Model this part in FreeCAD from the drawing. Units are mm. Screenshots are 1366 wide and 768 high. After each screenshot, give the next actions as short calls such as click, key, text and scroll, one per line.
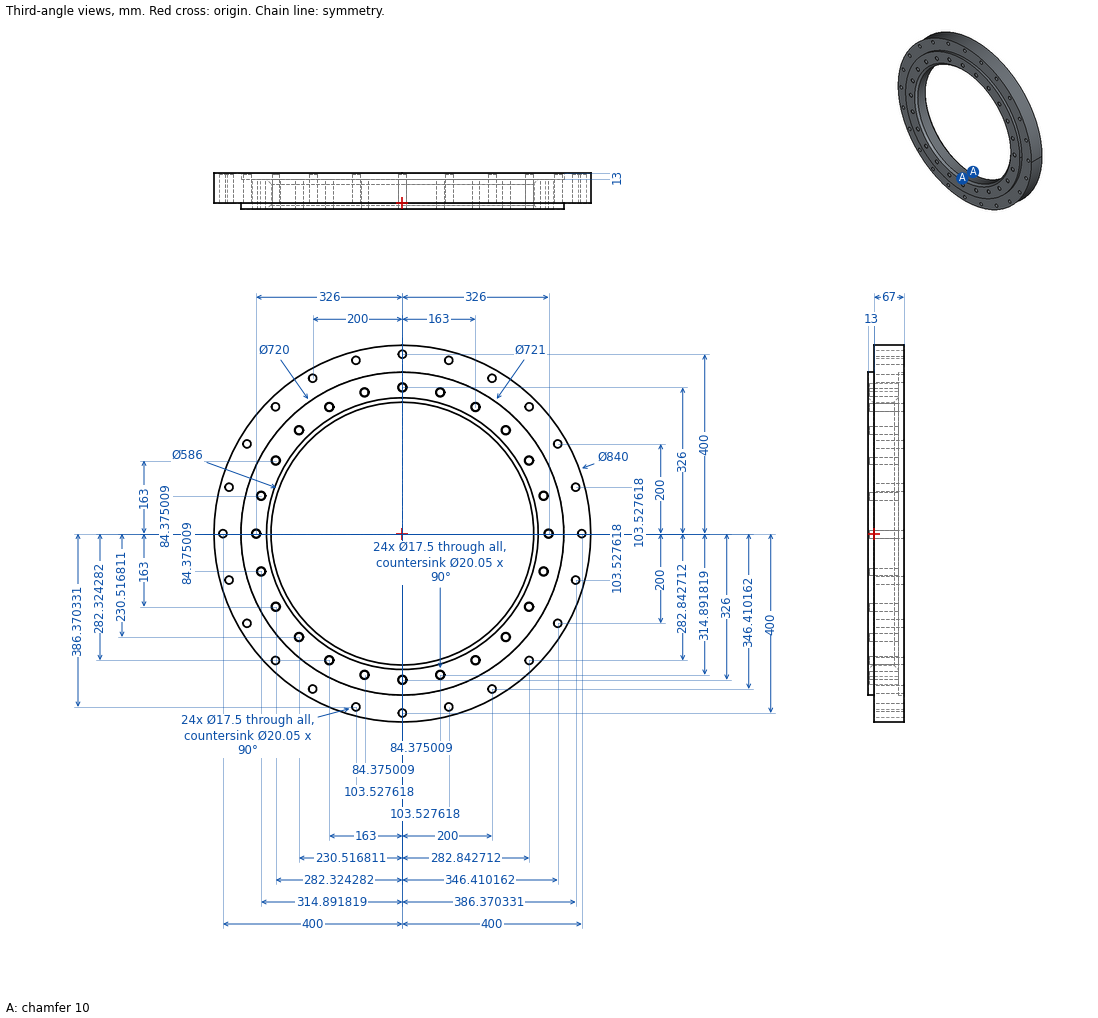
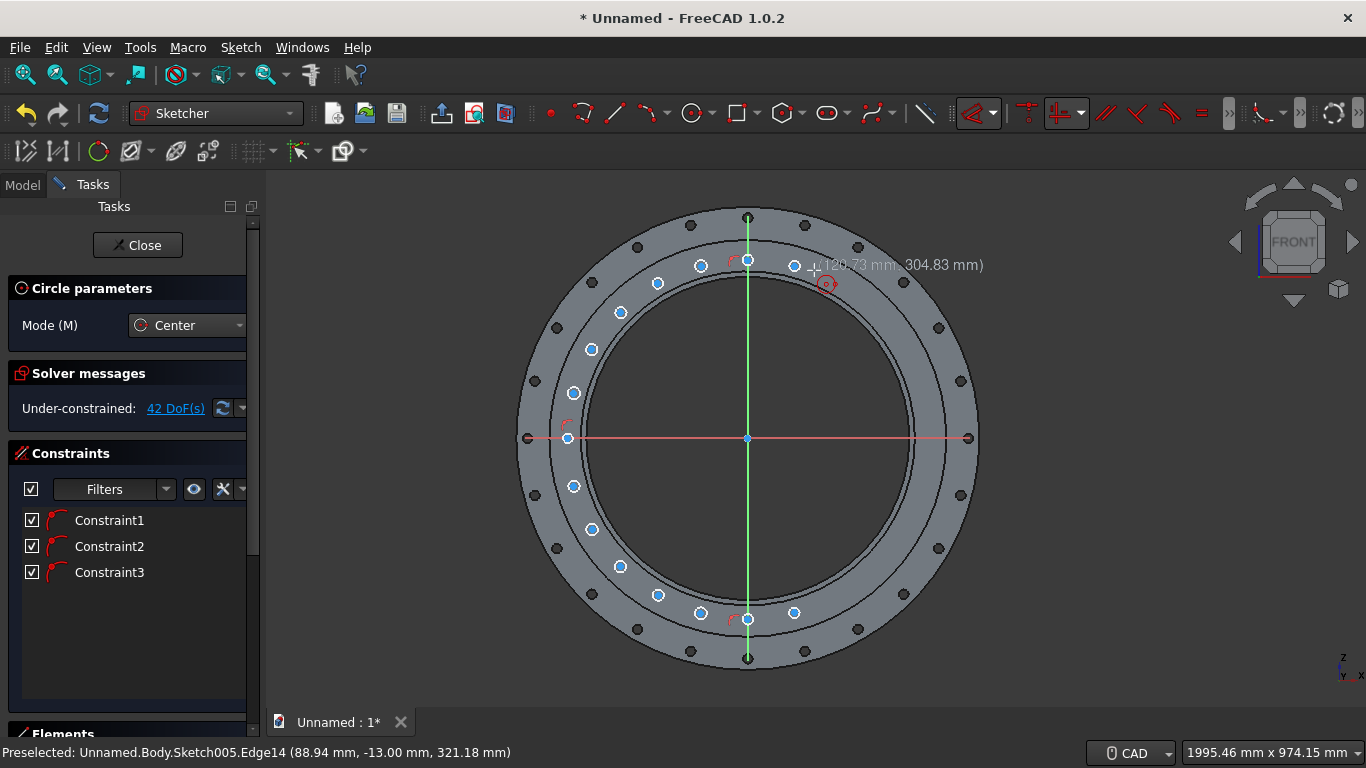
click(838, 283)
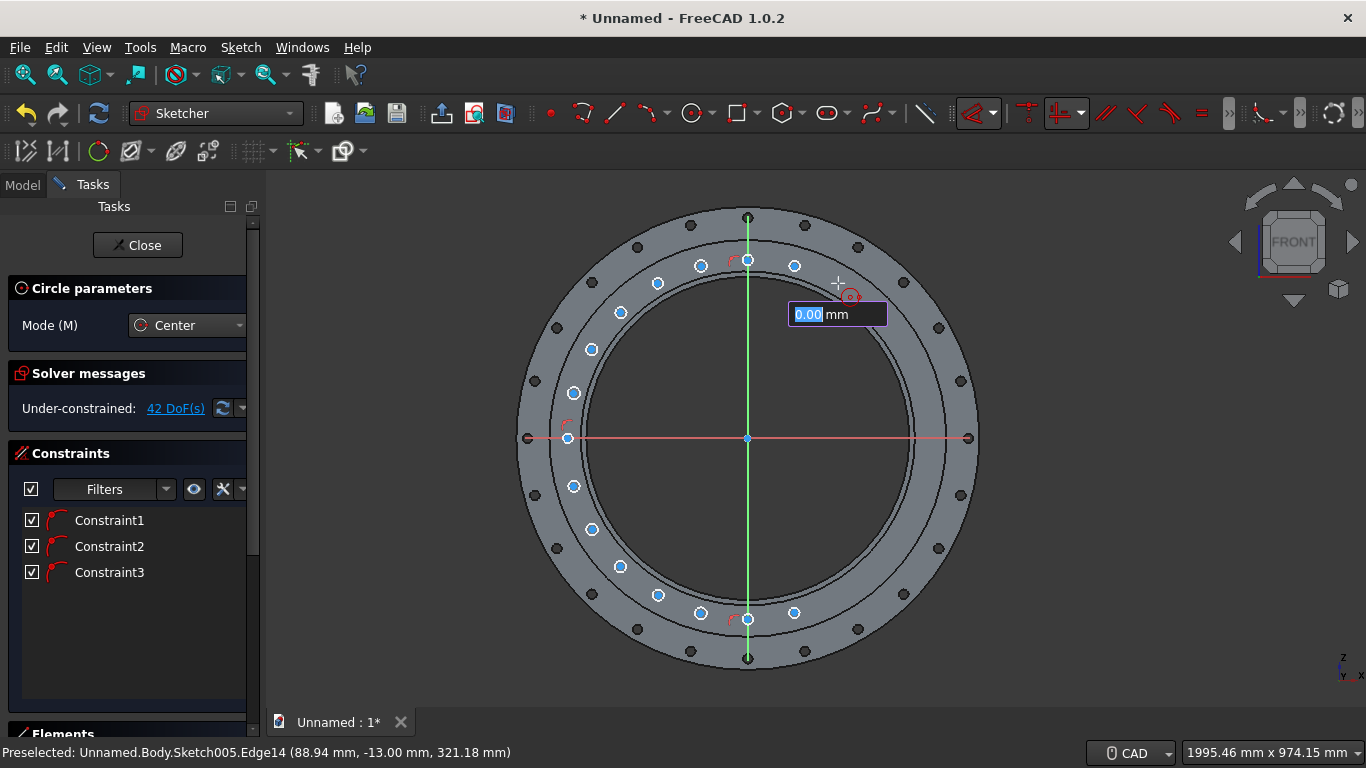
scroll(841, 279, up, 6)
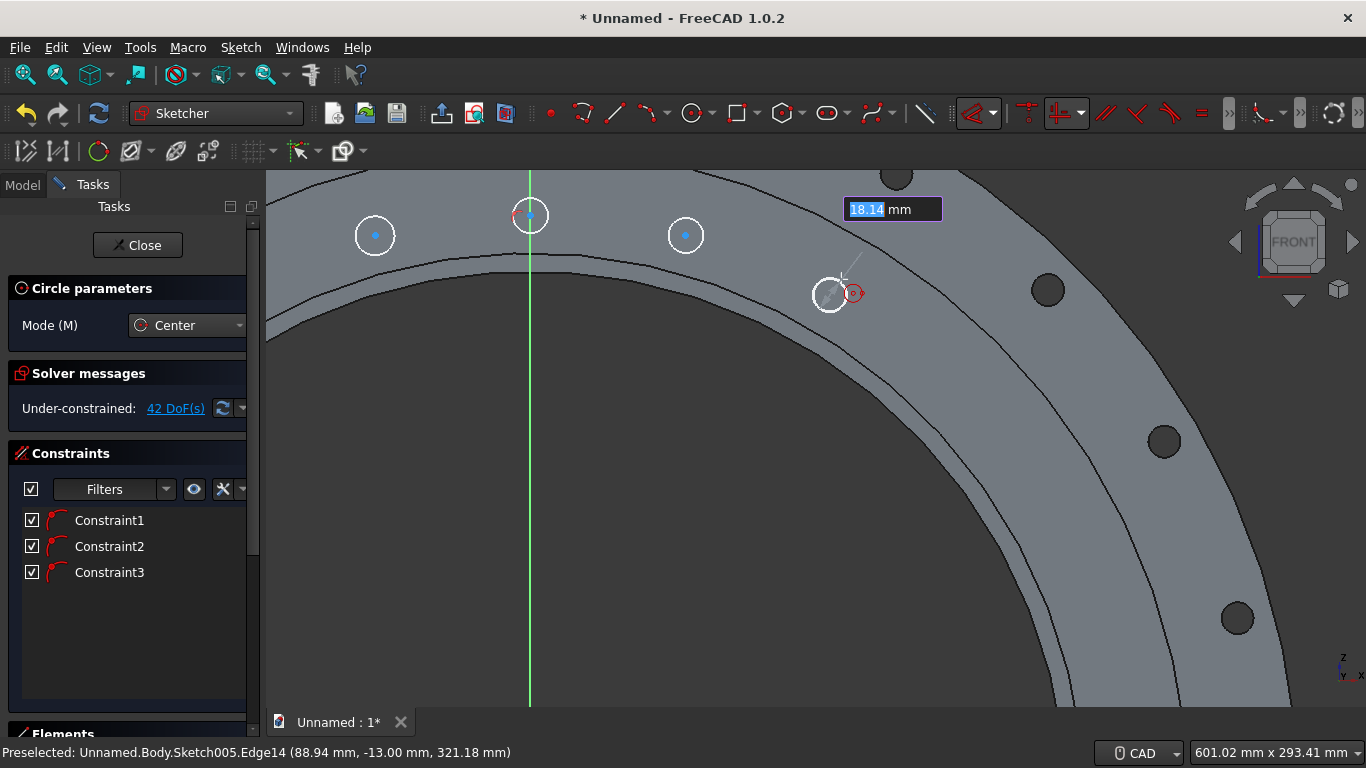
click(840, 280)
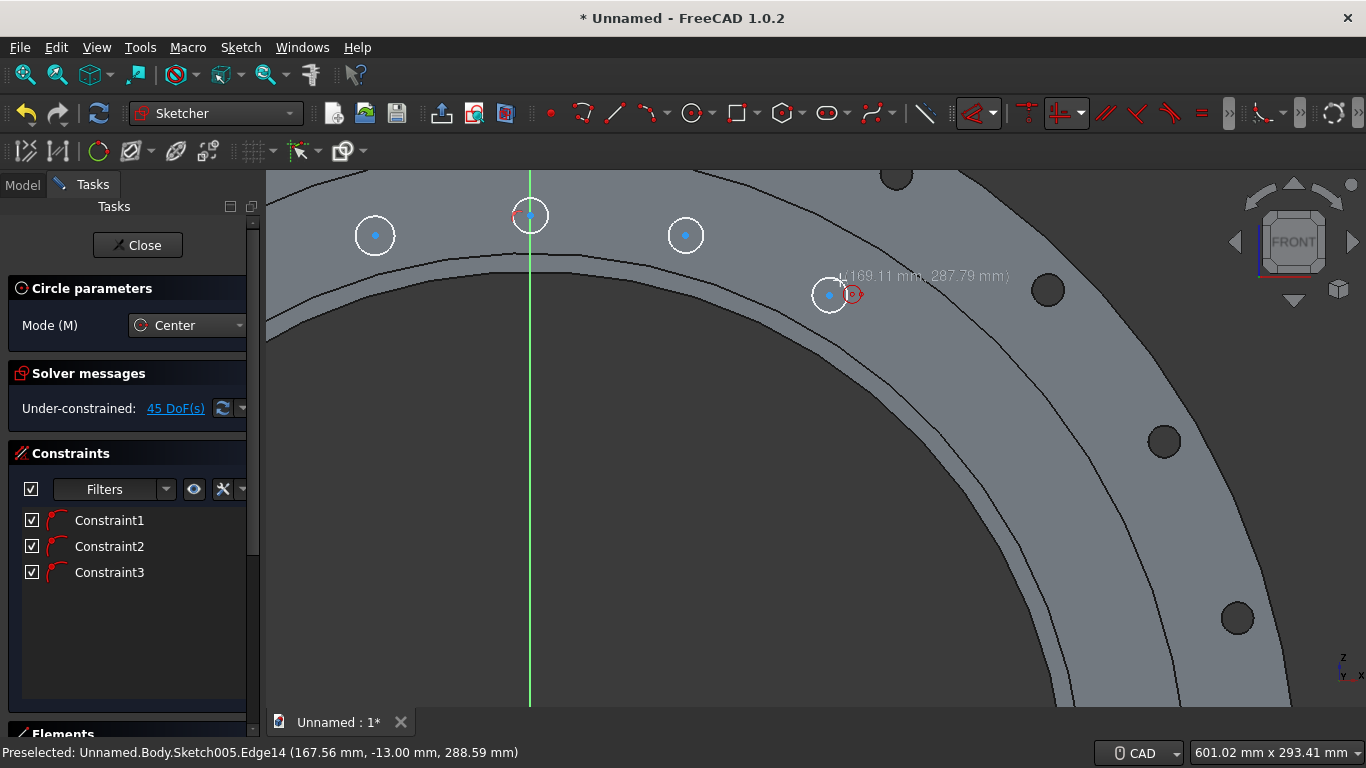
scroll(952, 386, up, 2)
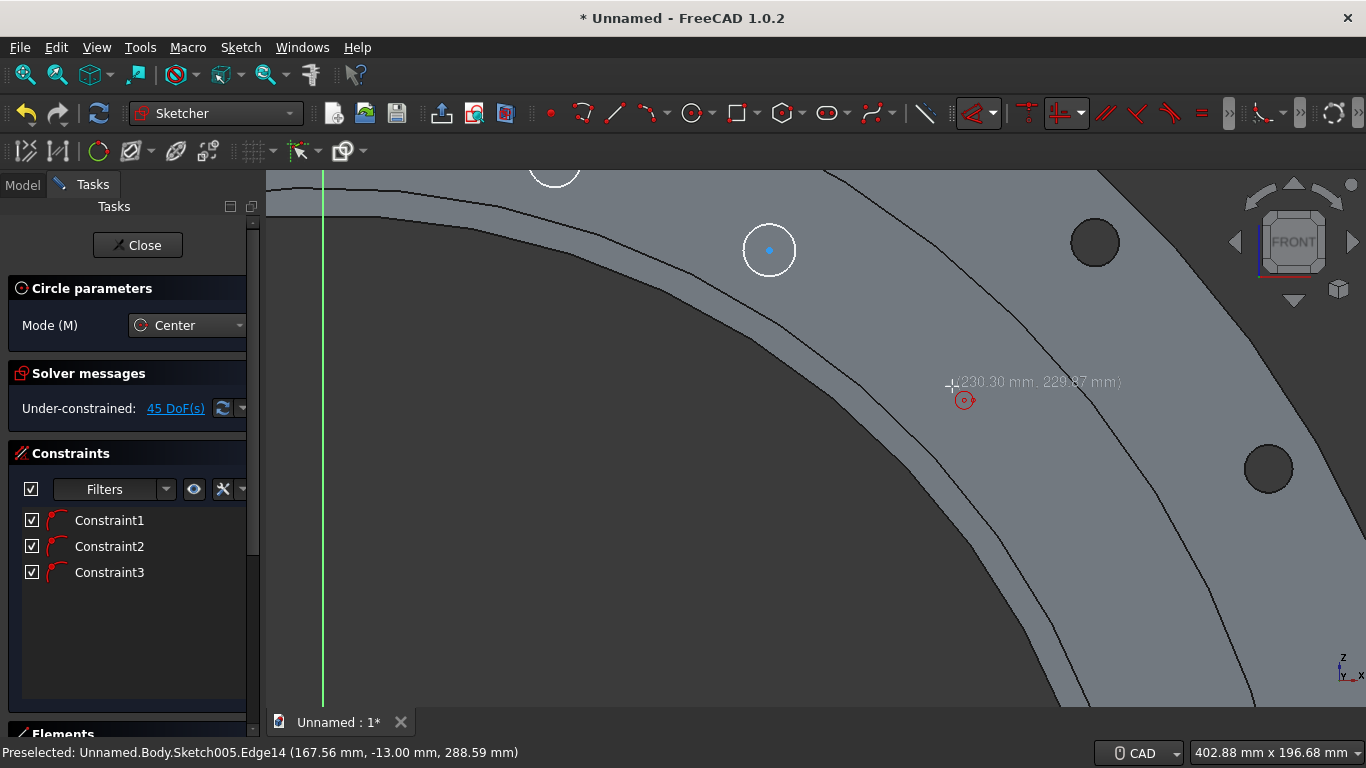
scroll(855, 293, down, 8)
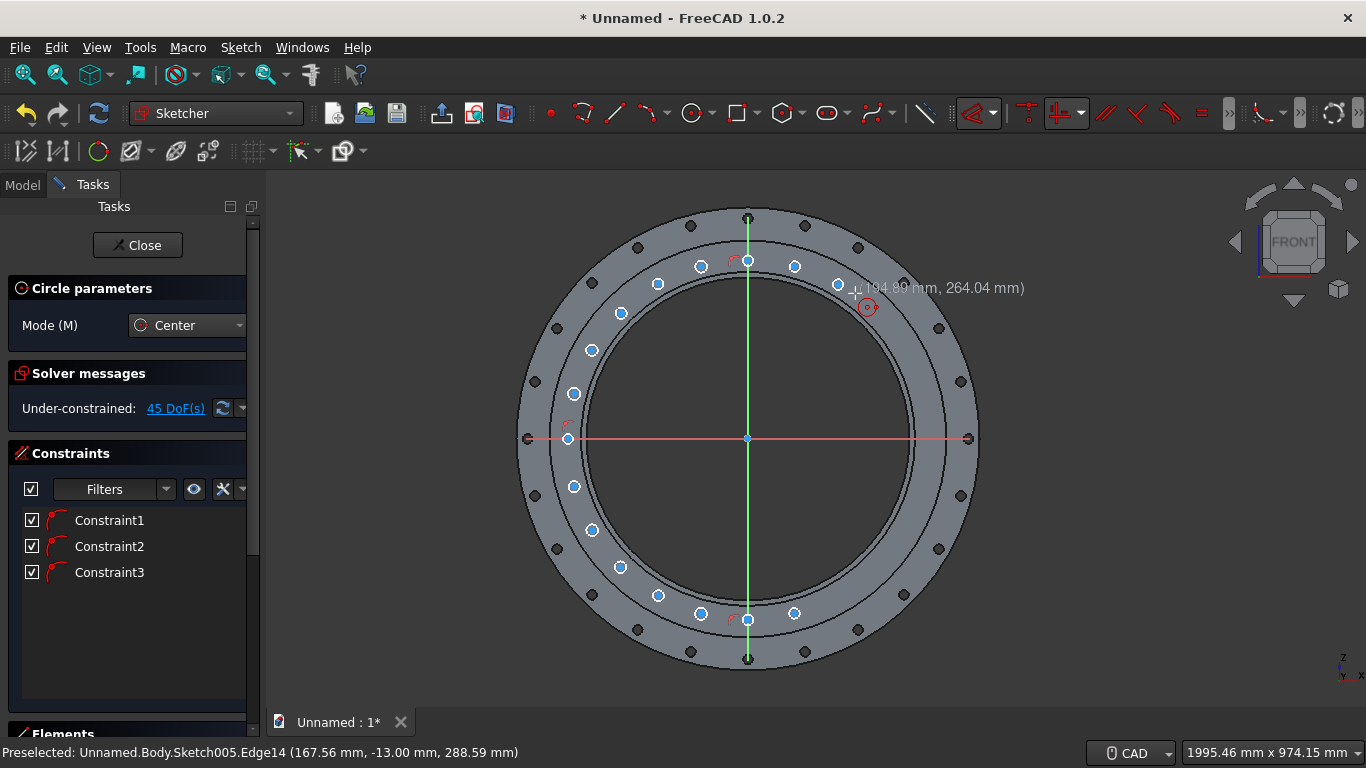
click(875, 312)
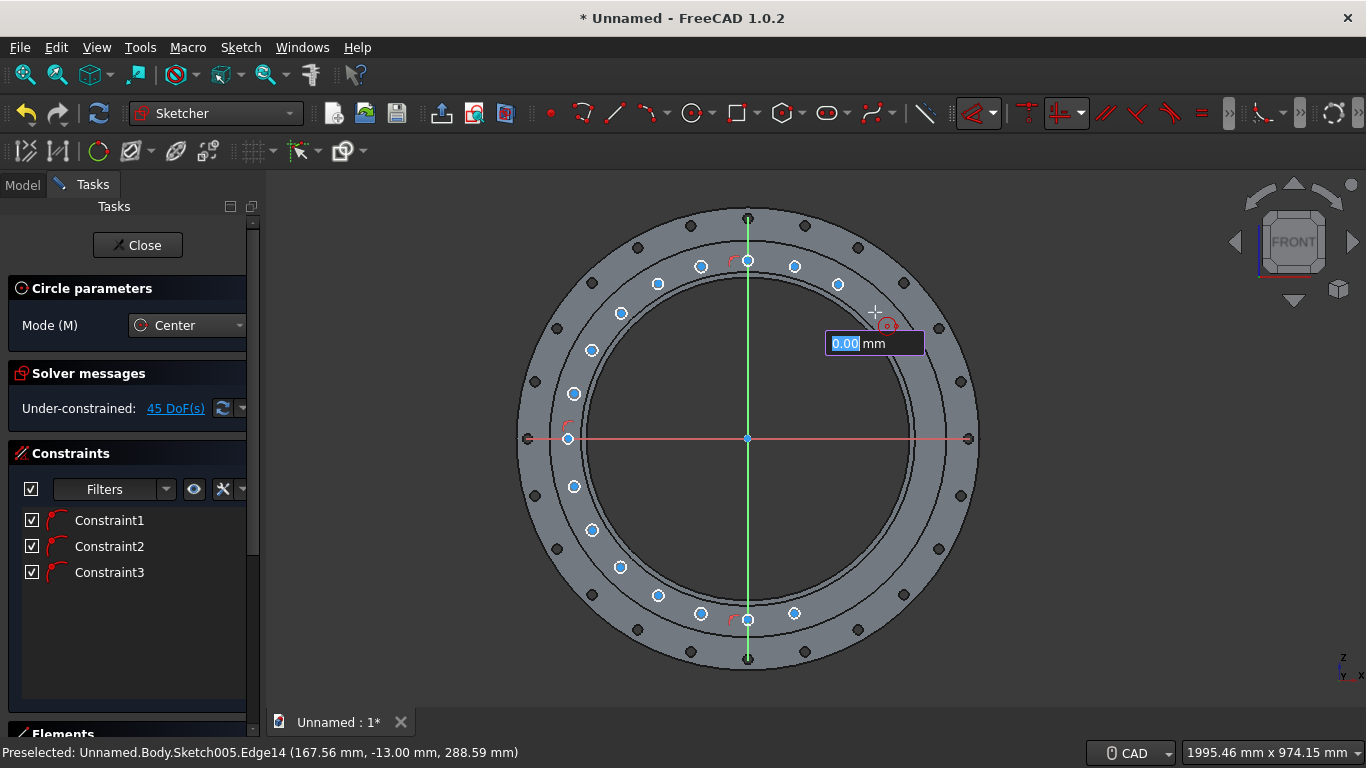
scroll(878, 308, up, 6)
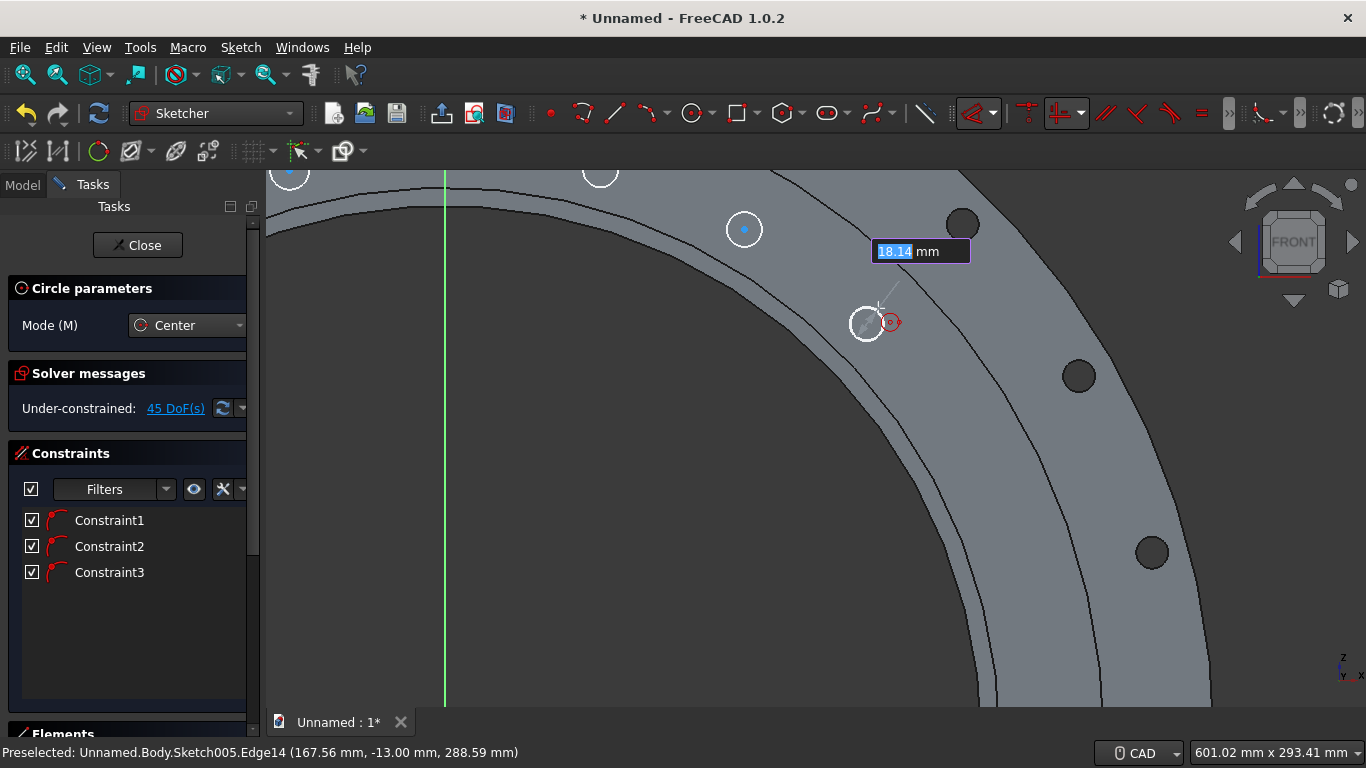
click(878, 309)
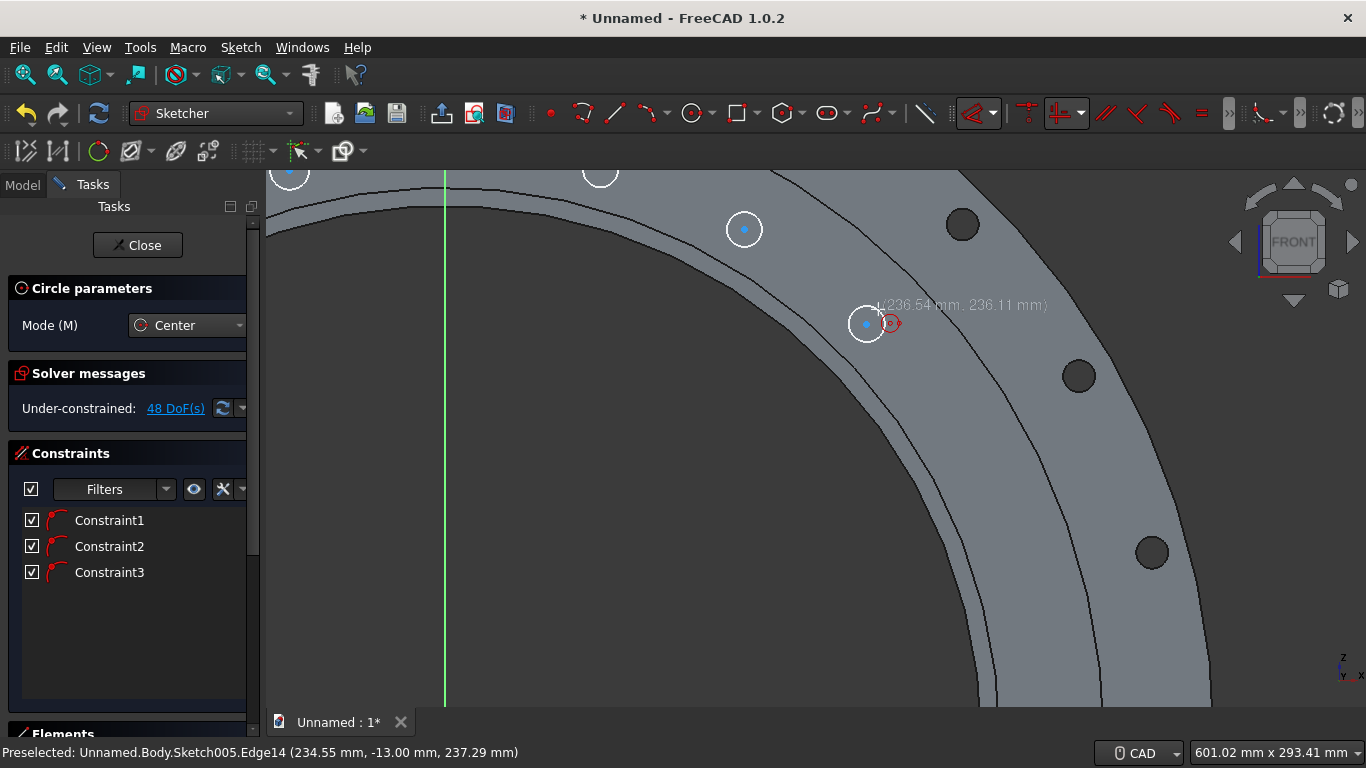
scroll(962, 444, up, 2)